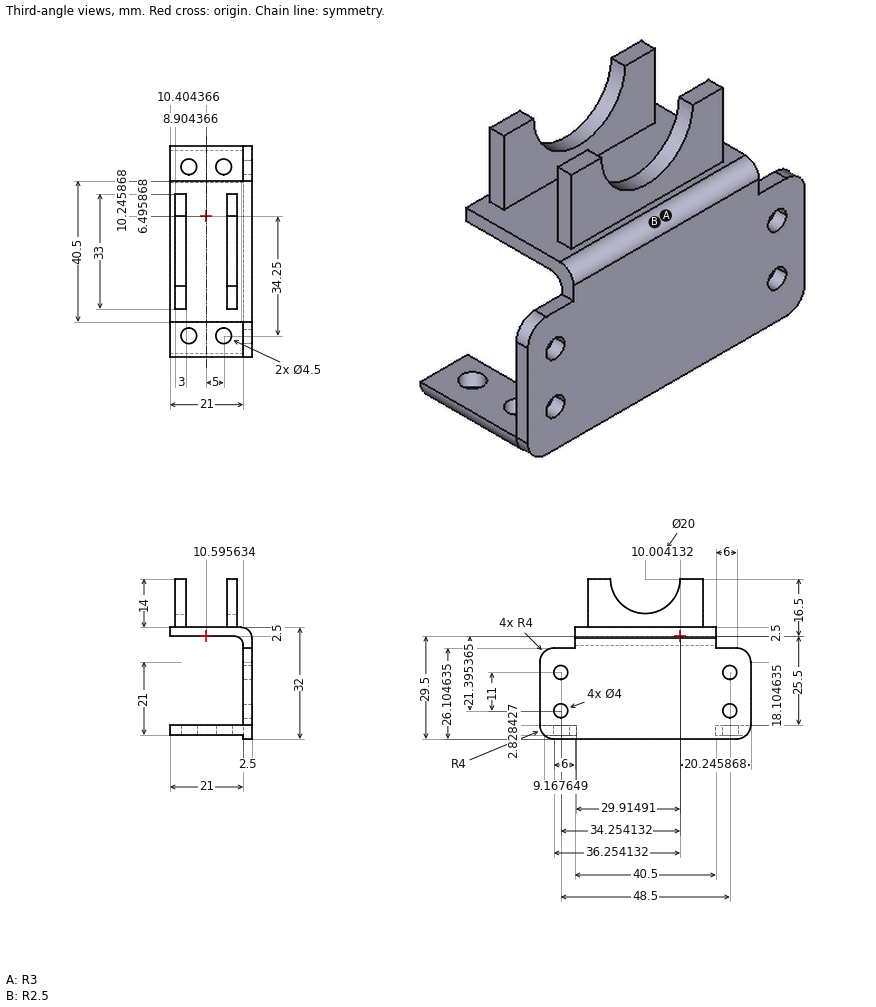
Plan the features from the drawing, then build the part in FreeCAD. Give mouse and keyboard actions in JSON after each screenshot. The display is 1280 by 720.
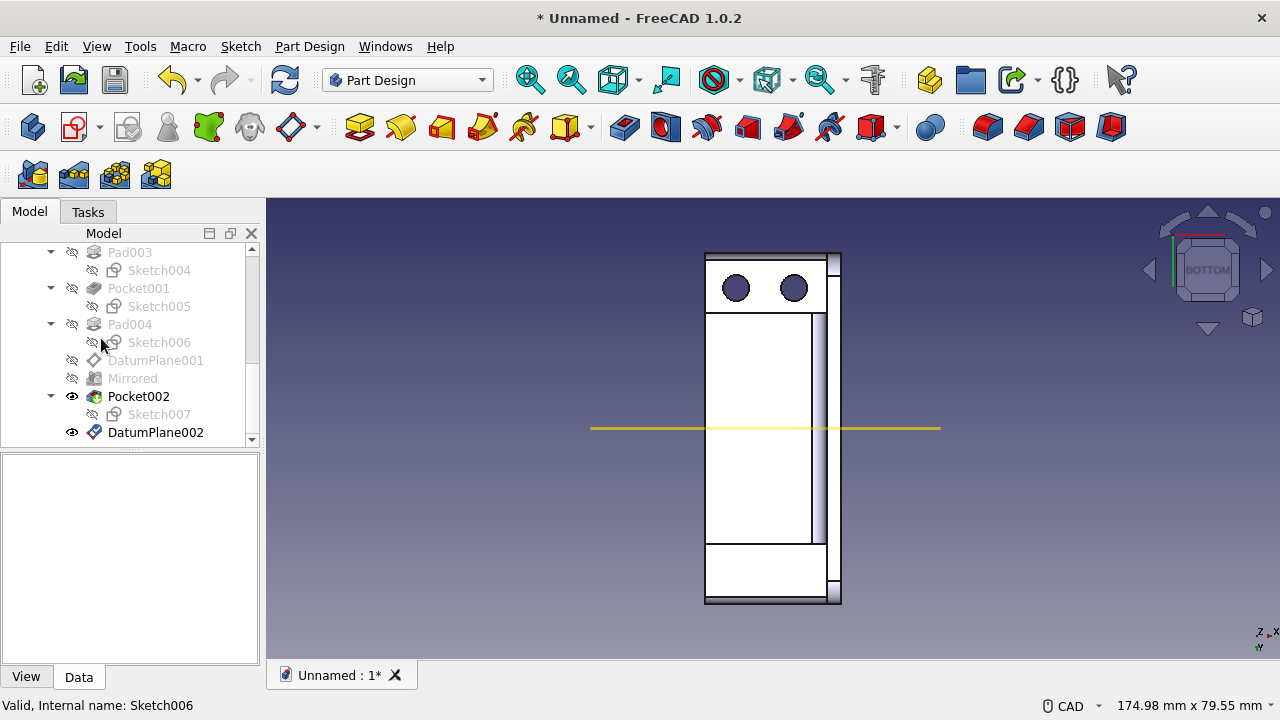
{"action": "left_click", "coordinate": [117, 396]}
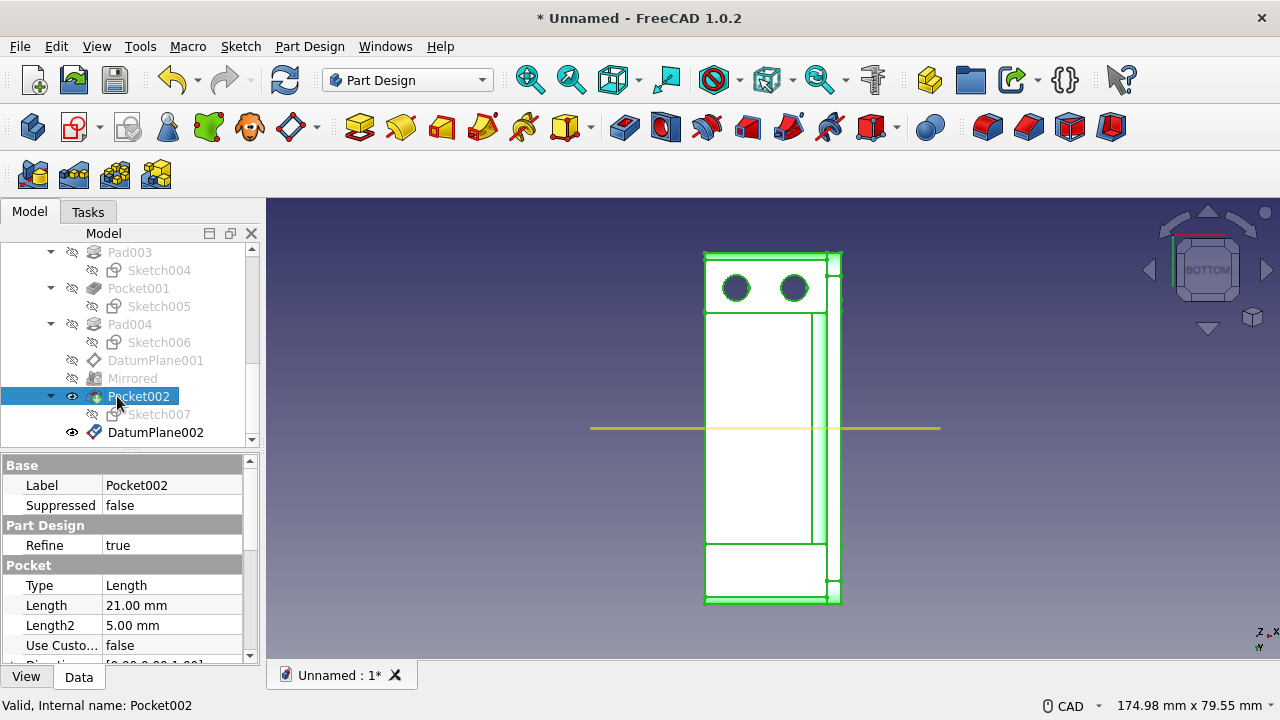
{"action": "left_click", "coordinate": [33, 174]}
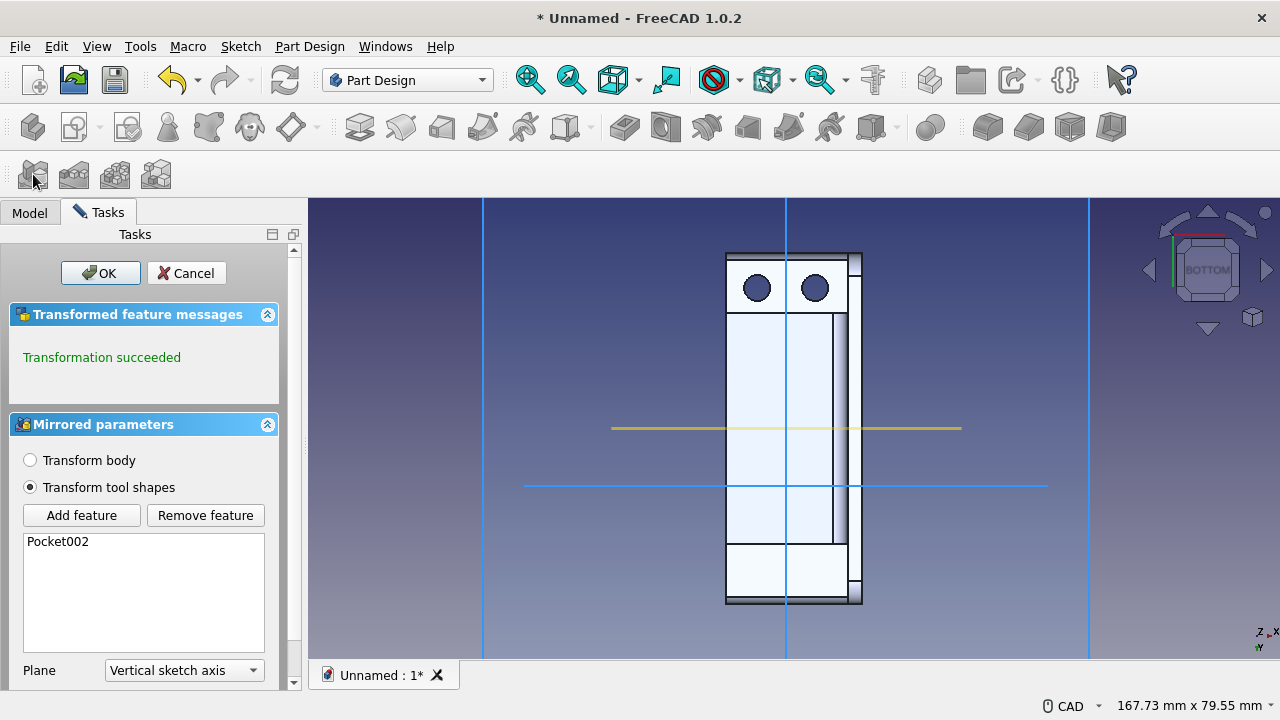
{"action": "left_click", "coordinate": [185, 670]}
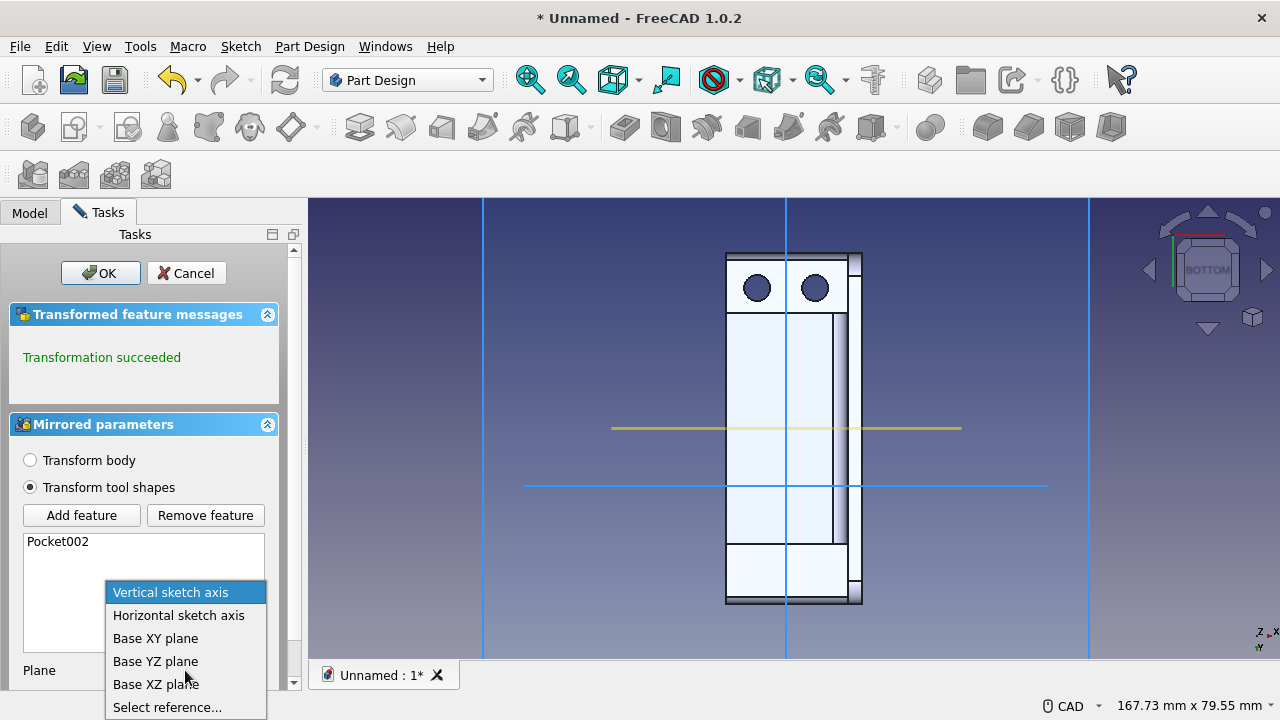
{"action": "left_click", "coordinate": [184, 708]}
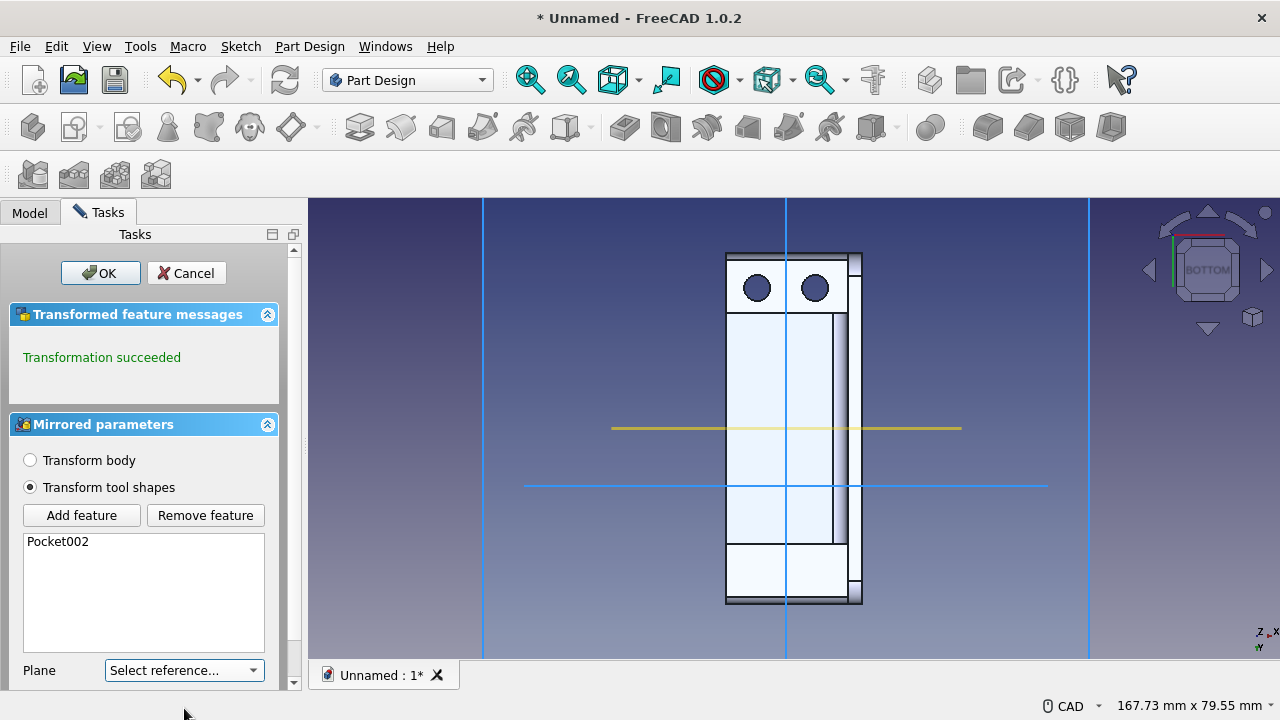
{"action": "left_click", "coordinate": [30, 212]}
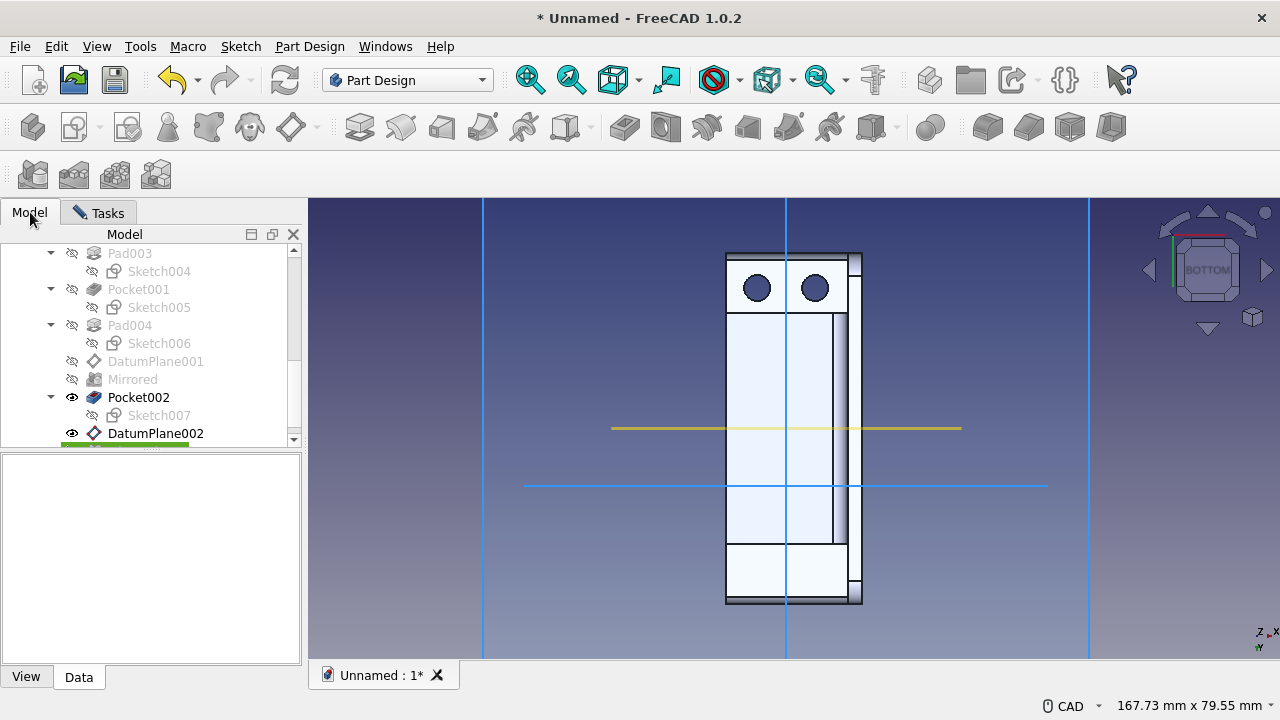
{"action": "left_click", "coordinate": [117, 433]}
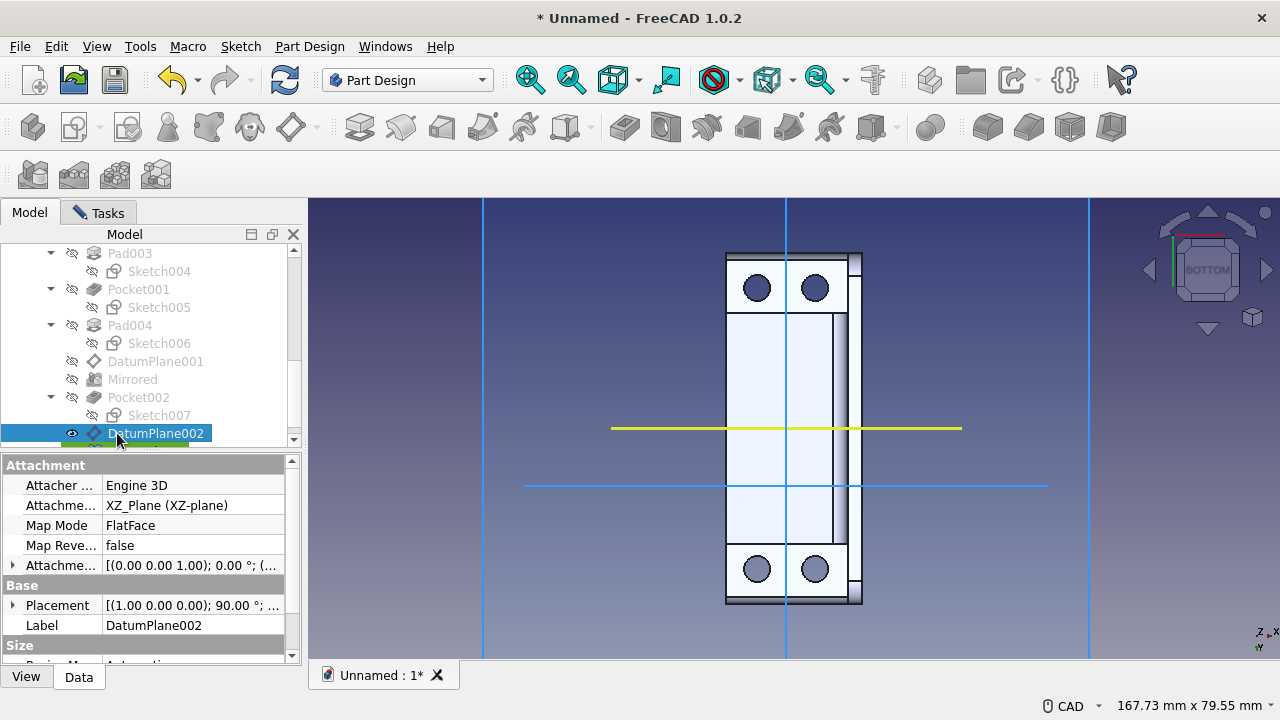
{"action": "left_click", "coordinate": [98, 212]}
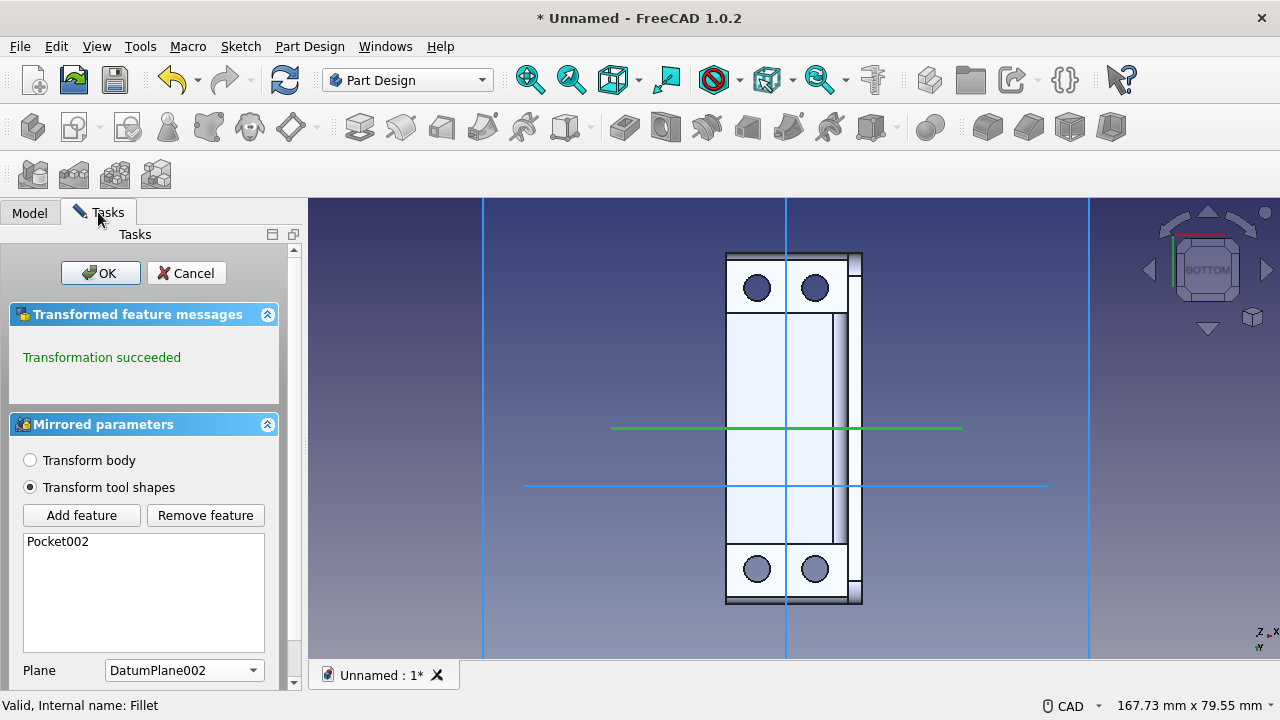
{"action": "left_click", "coordinate": [101, 273]}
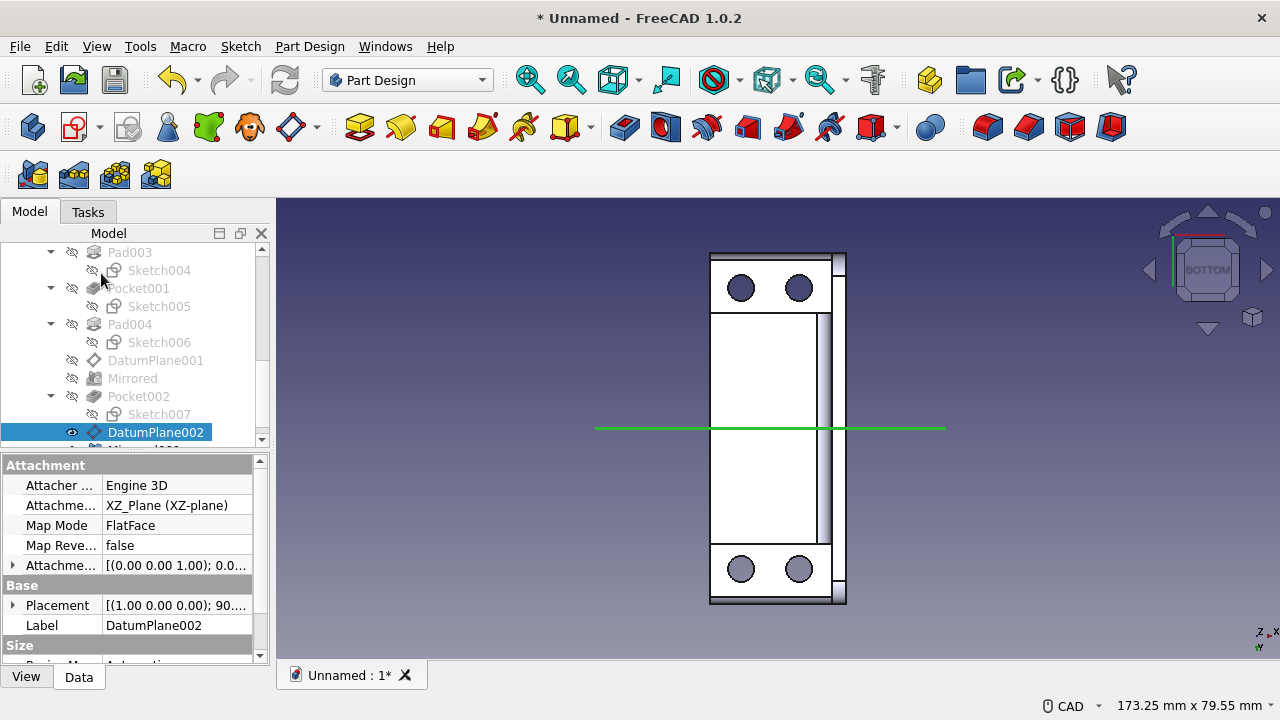
{"action": "left_click", "coordinate": [117, 432]}
{"action": "key", "text": "space"}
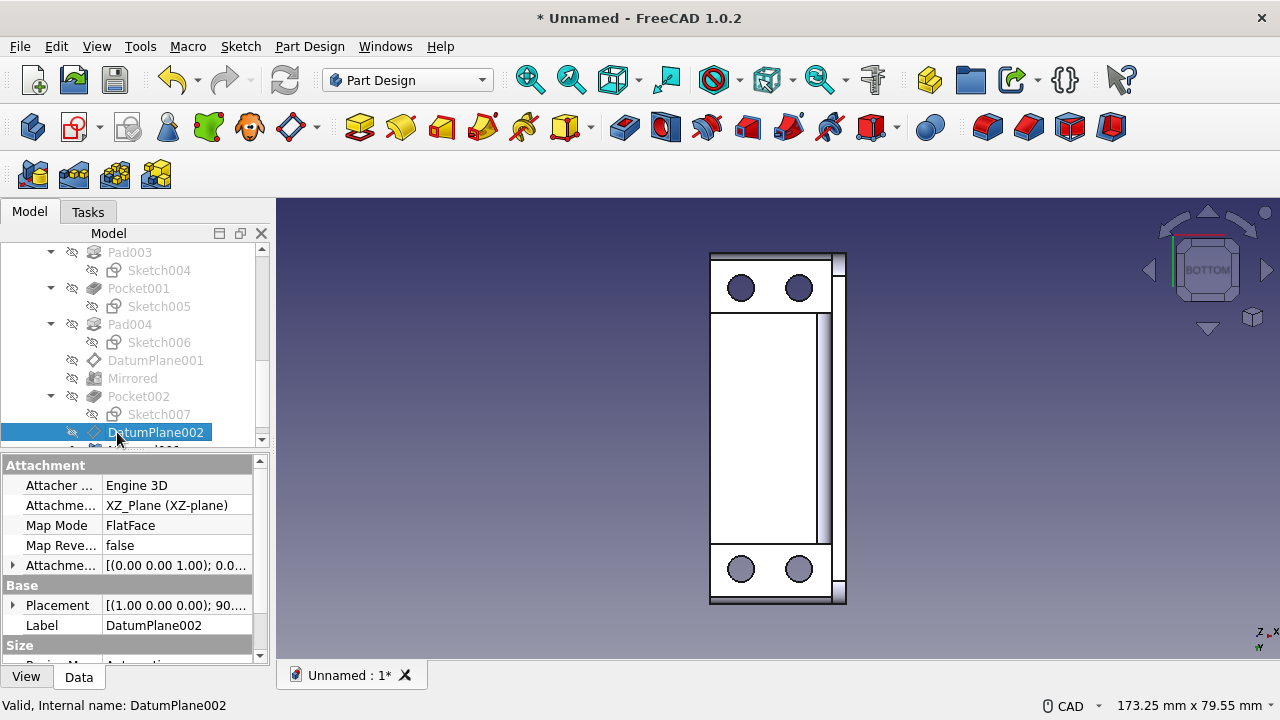
{"action": "key", "text": "0"}